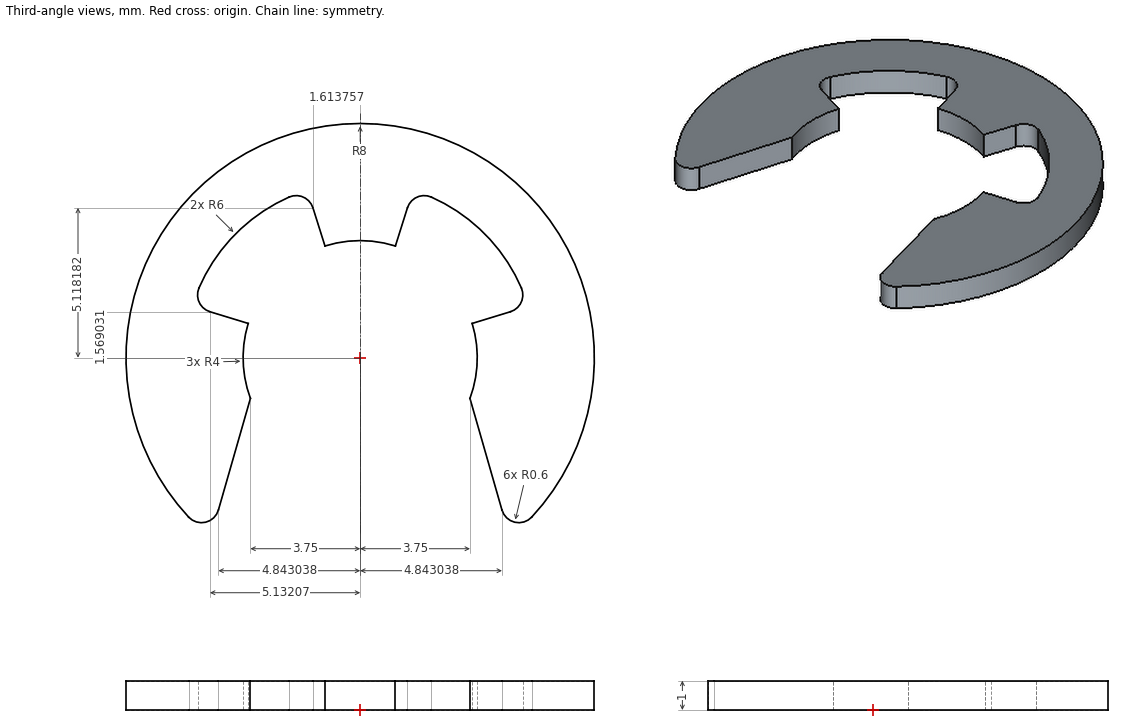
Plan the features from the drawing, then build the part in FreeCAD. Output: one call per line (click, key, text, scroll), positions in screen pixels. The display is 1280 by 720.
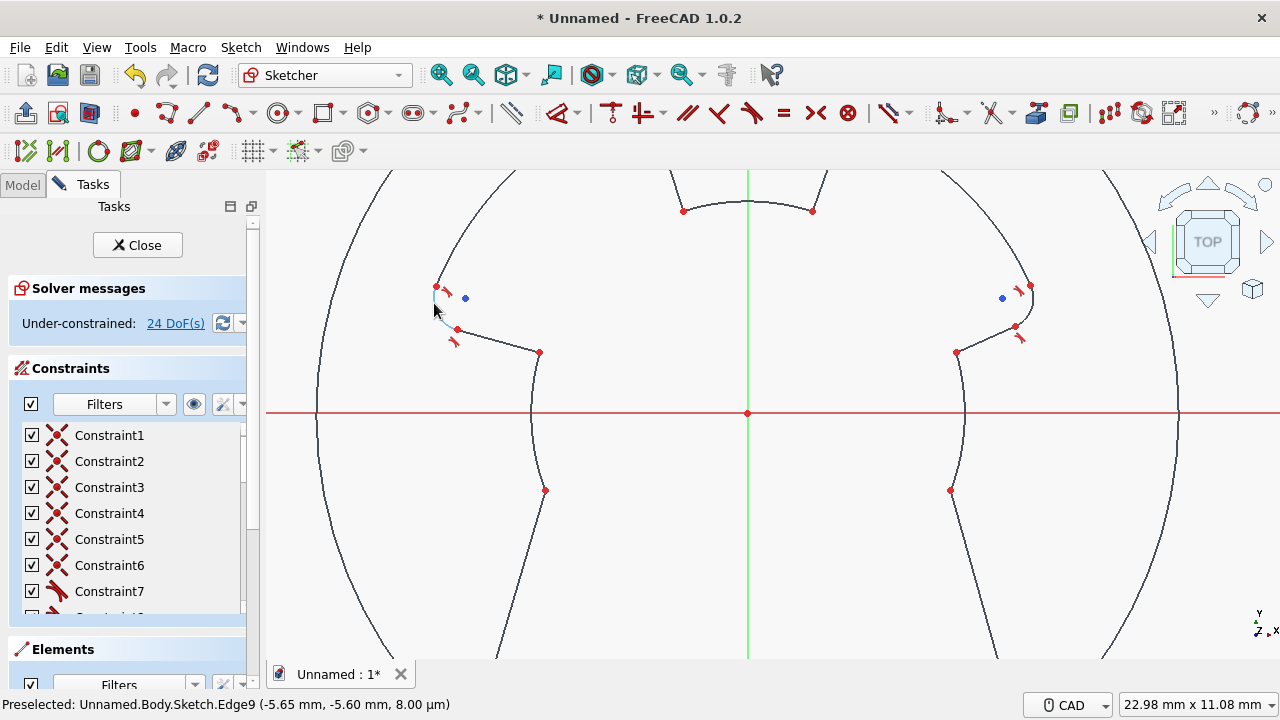
click(434, 303)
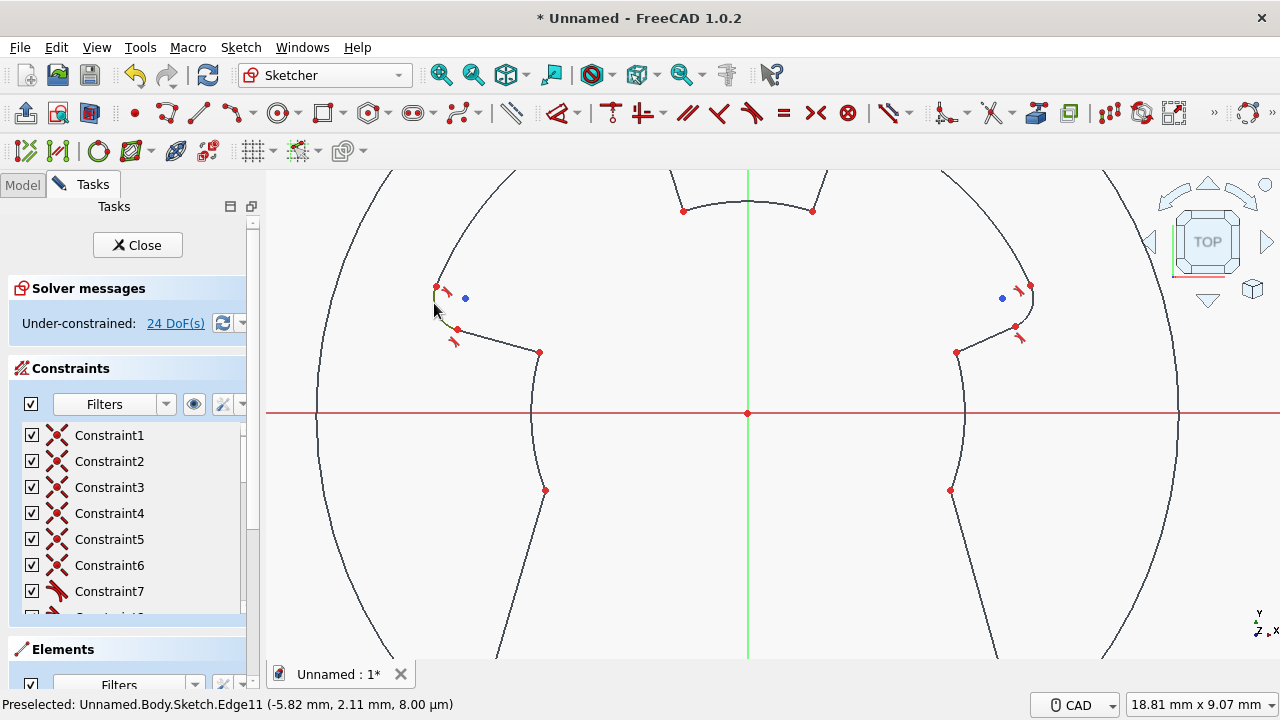
scroll(669, 468, down, 4)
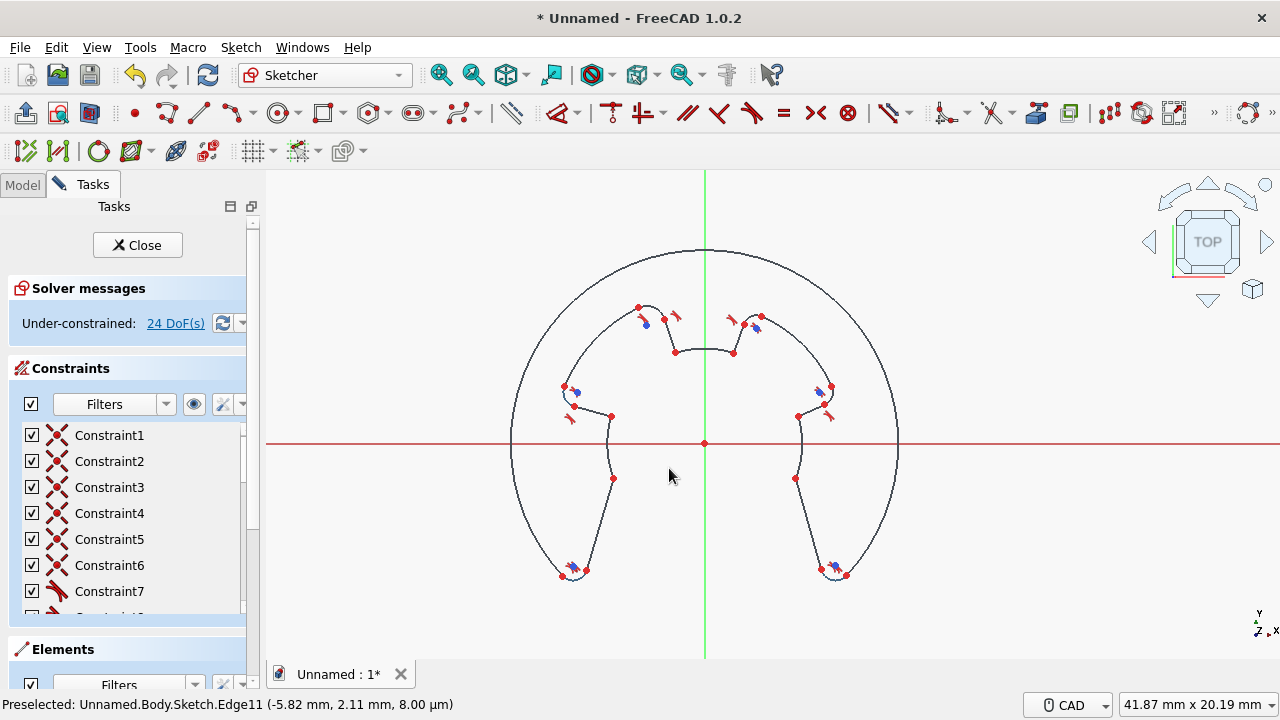
scroll(660, 311, up, 2)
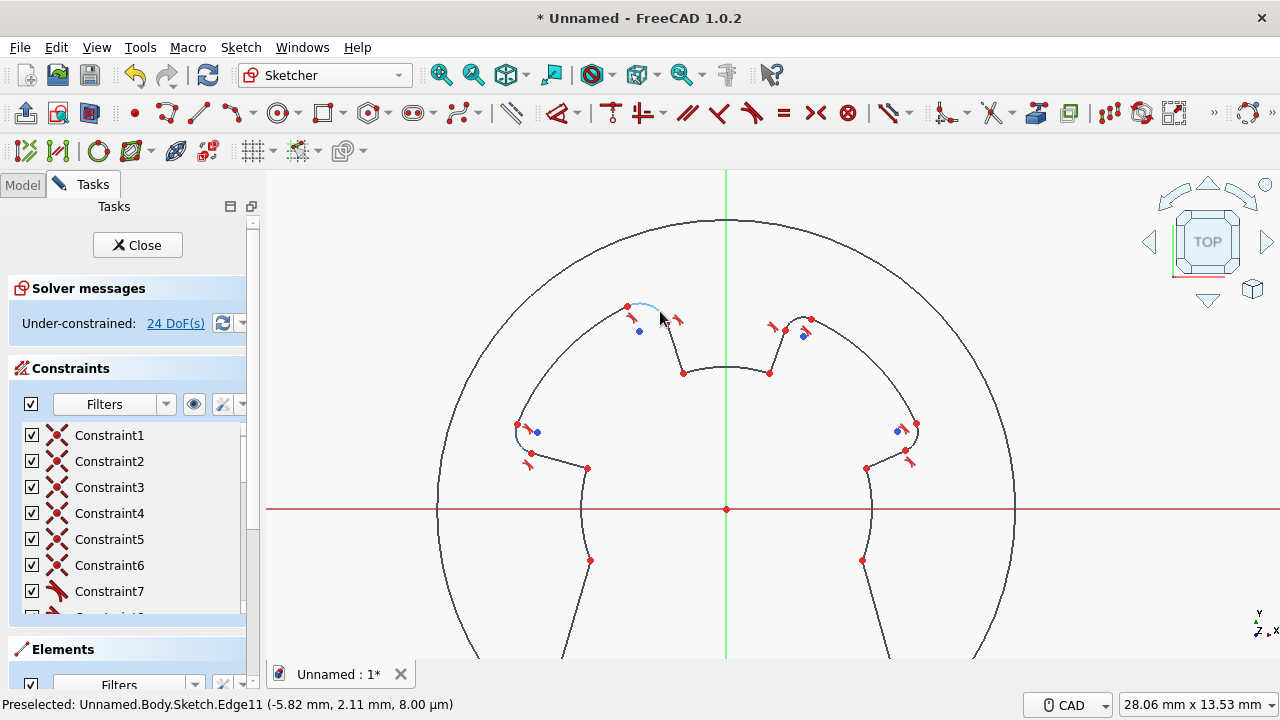
click(659, 311)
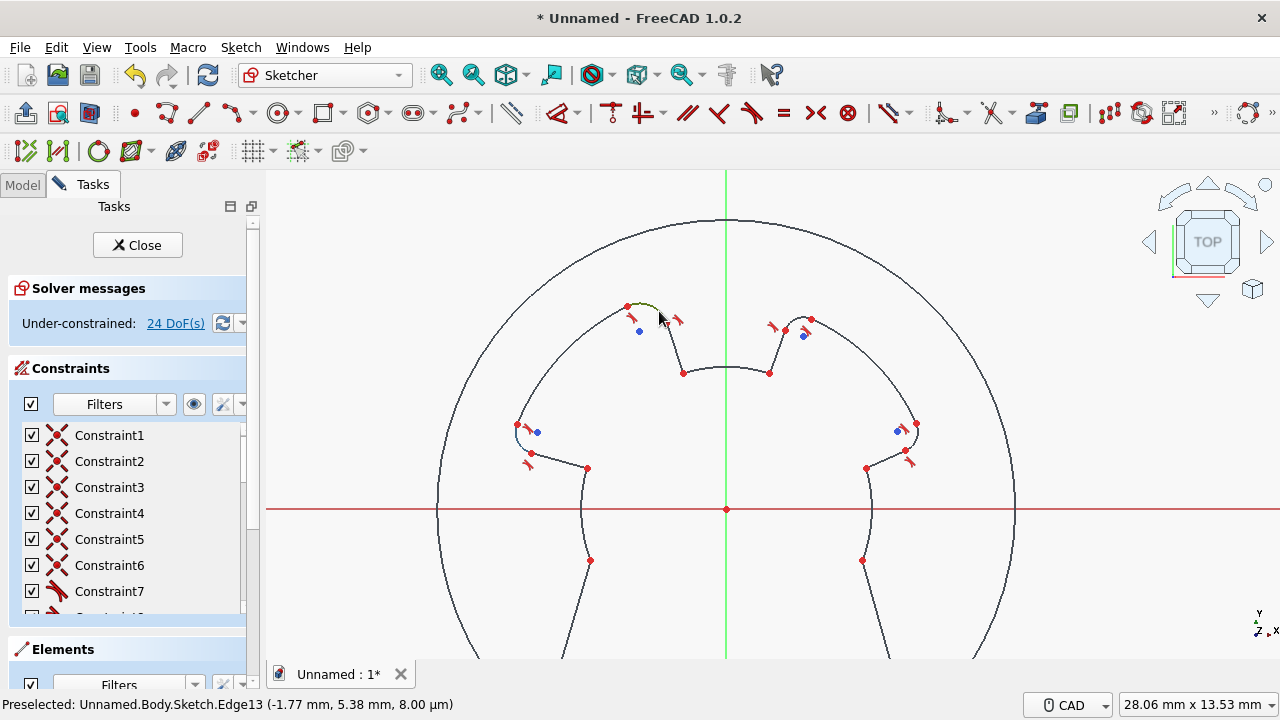
scroll(802, 317, up, 2)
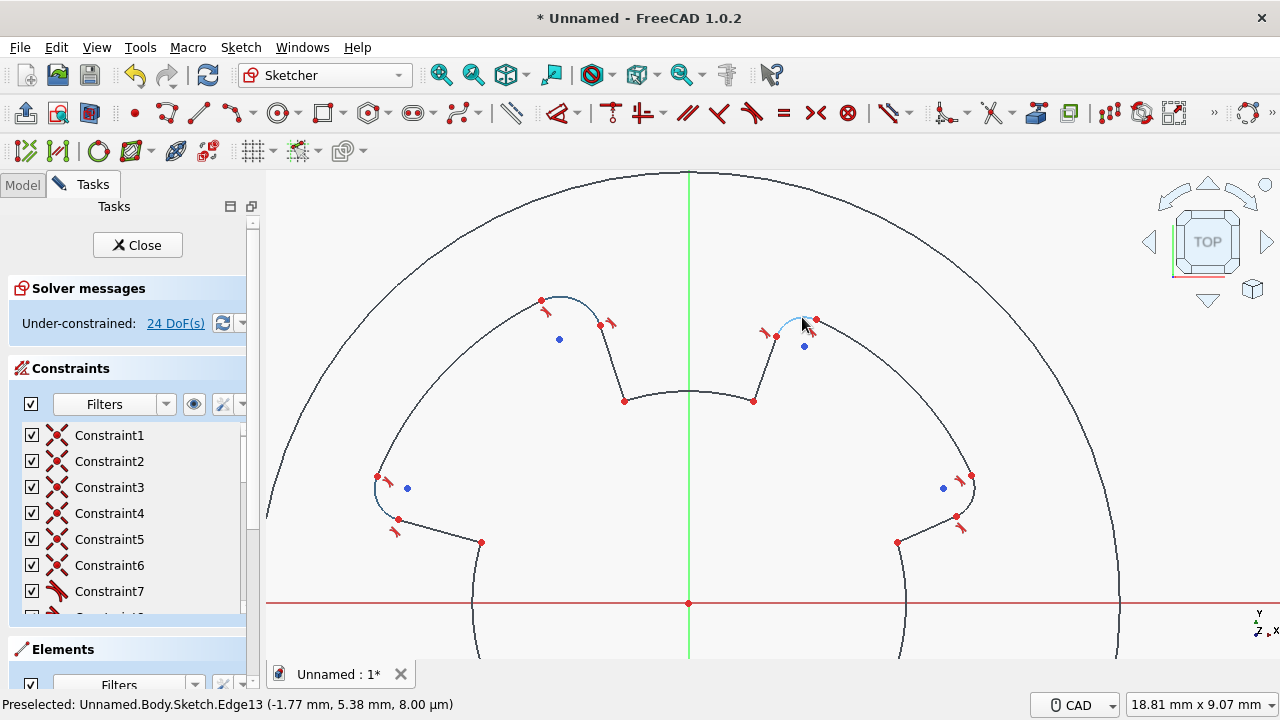
click(802, 317)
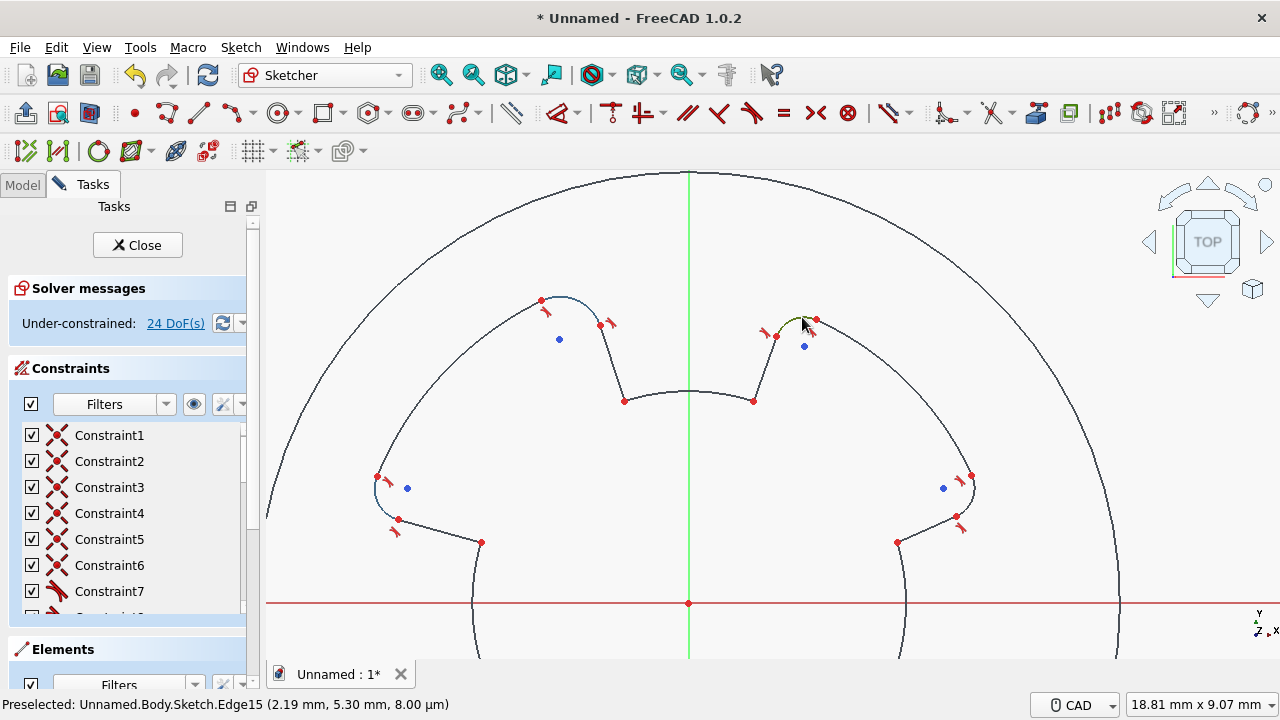
click(968, 508)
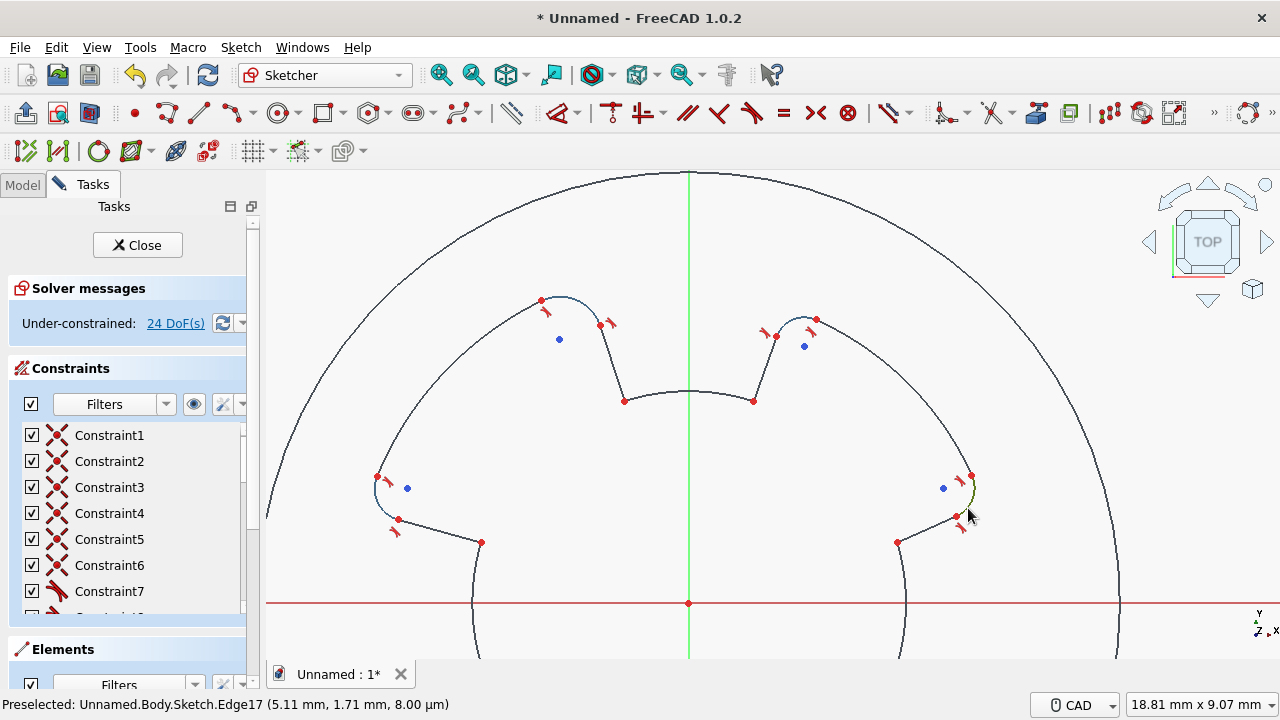
key(e)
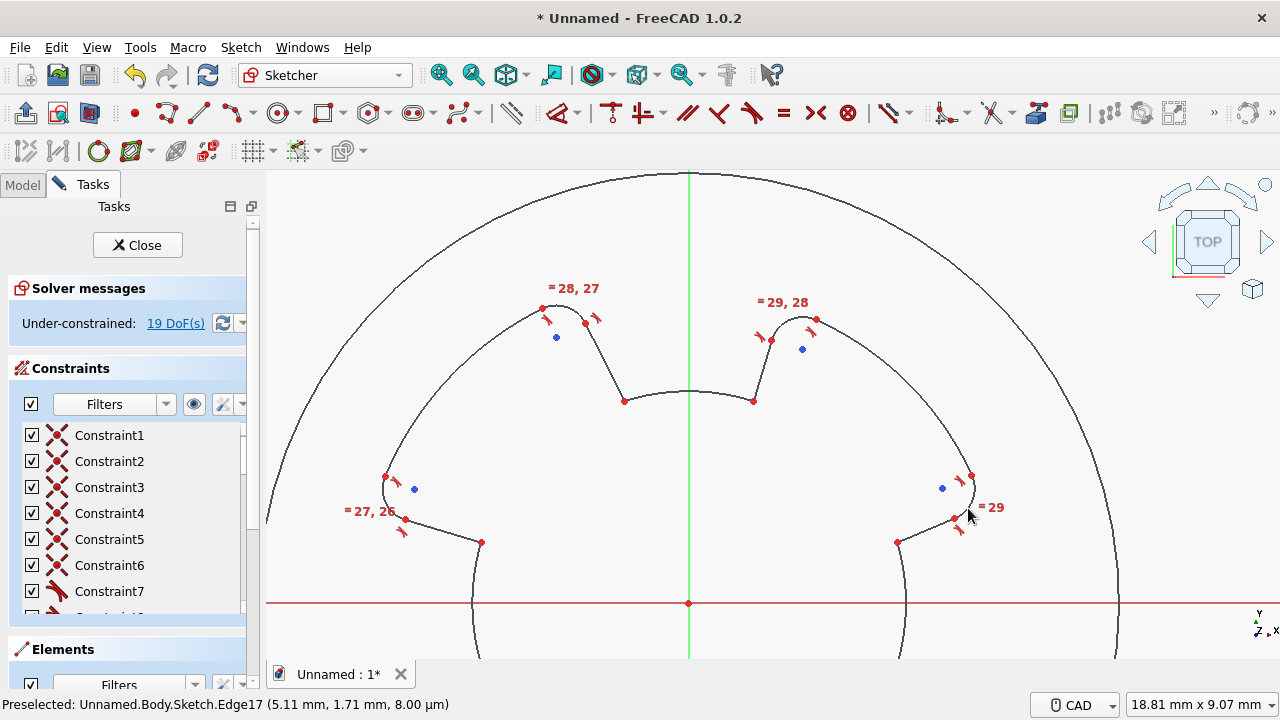
click(473, 584)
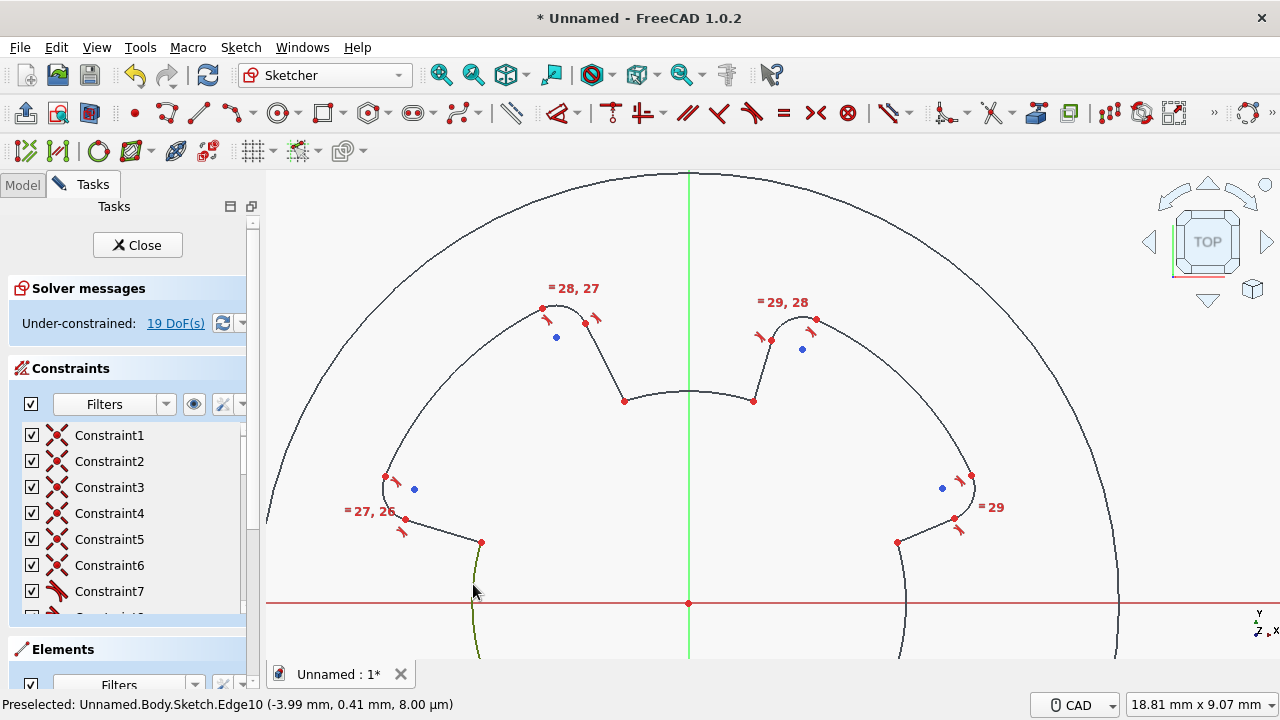
click(715, 393)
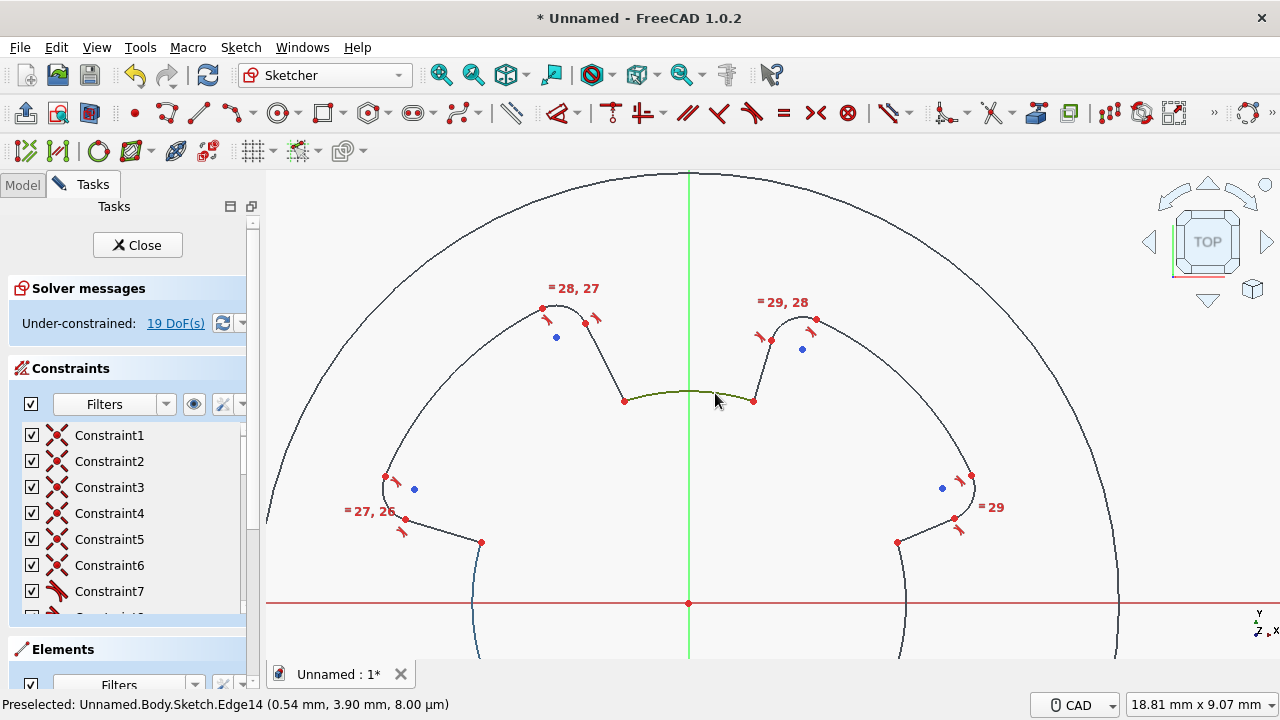
click(905, 584)